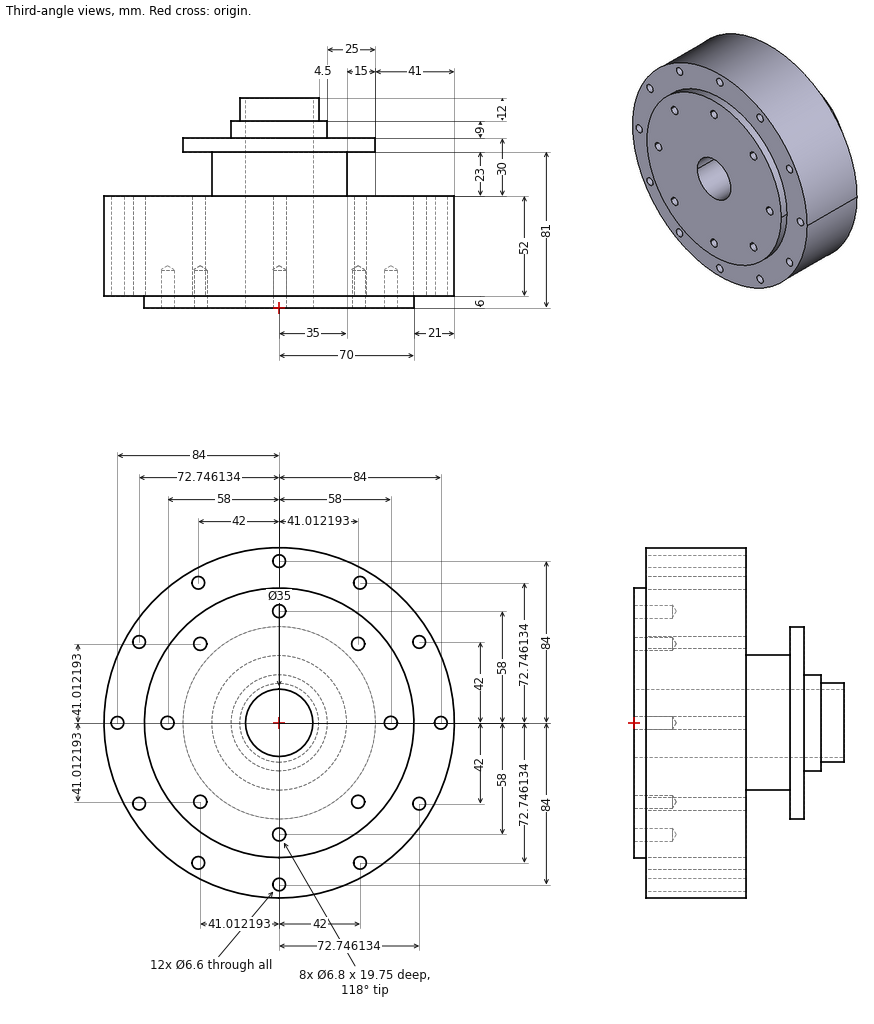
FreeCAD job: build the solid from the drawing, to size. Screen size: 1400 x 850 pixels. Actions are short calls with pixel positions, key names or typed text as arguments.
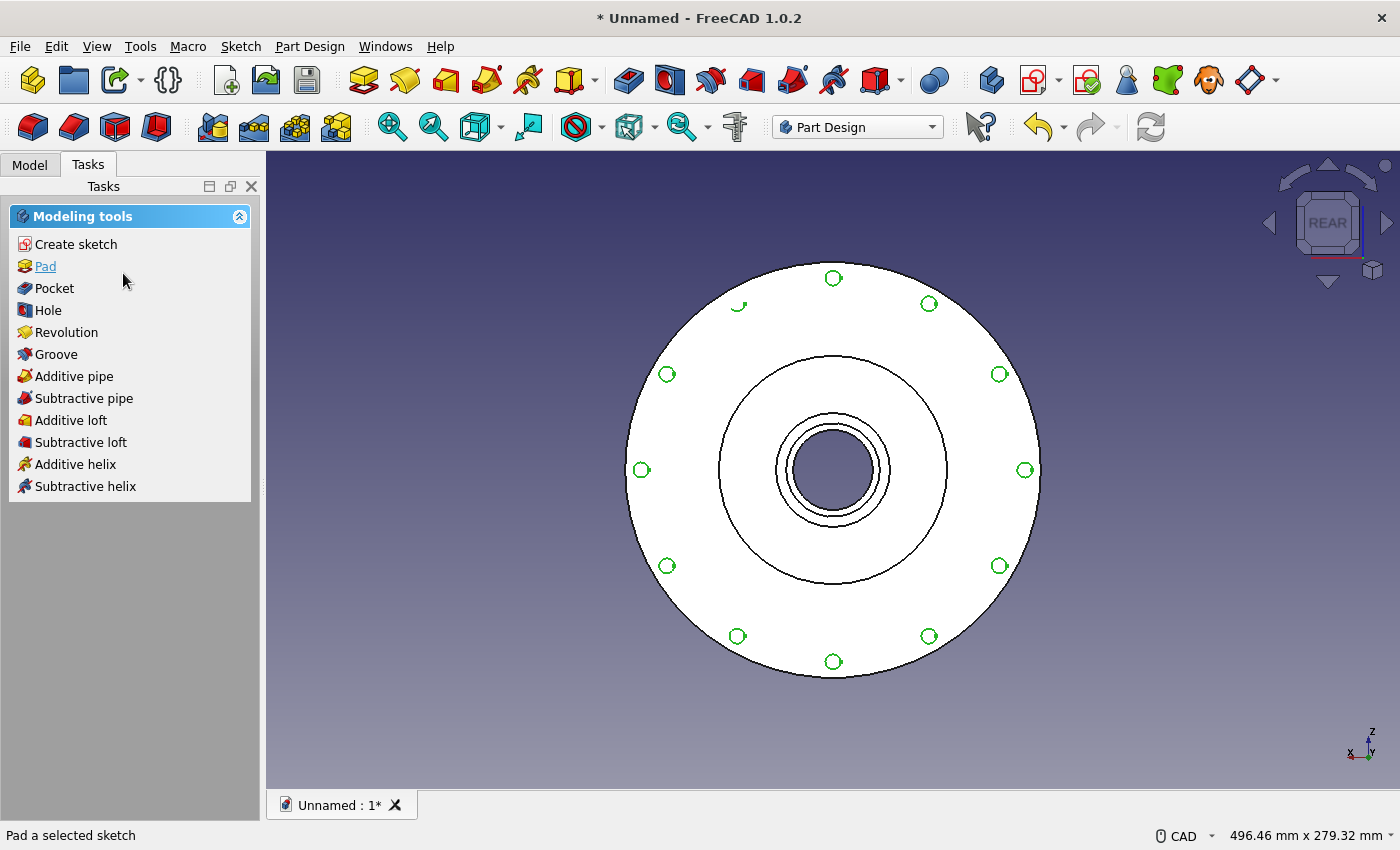
click(670, 80)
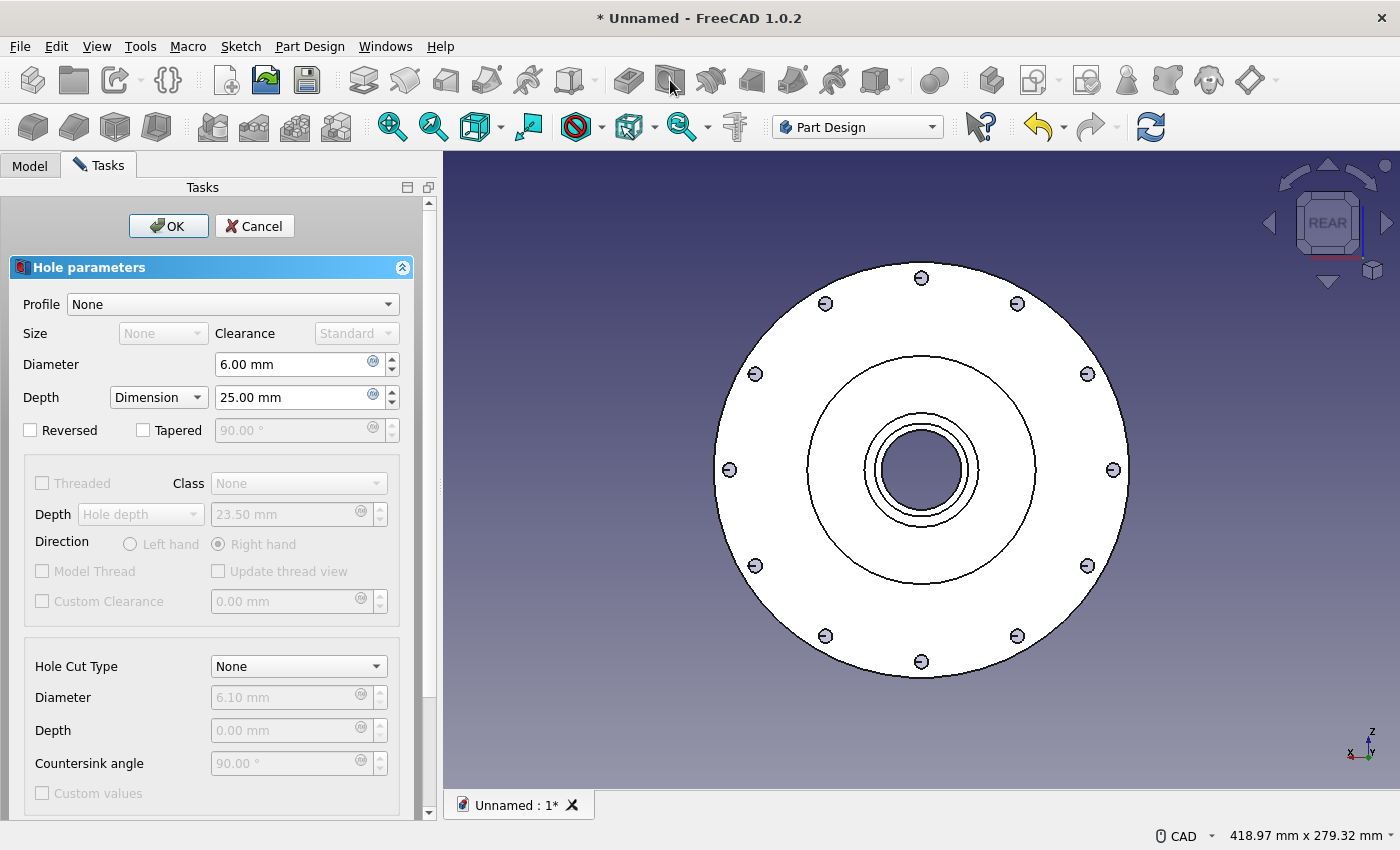
triple_click(300, 364)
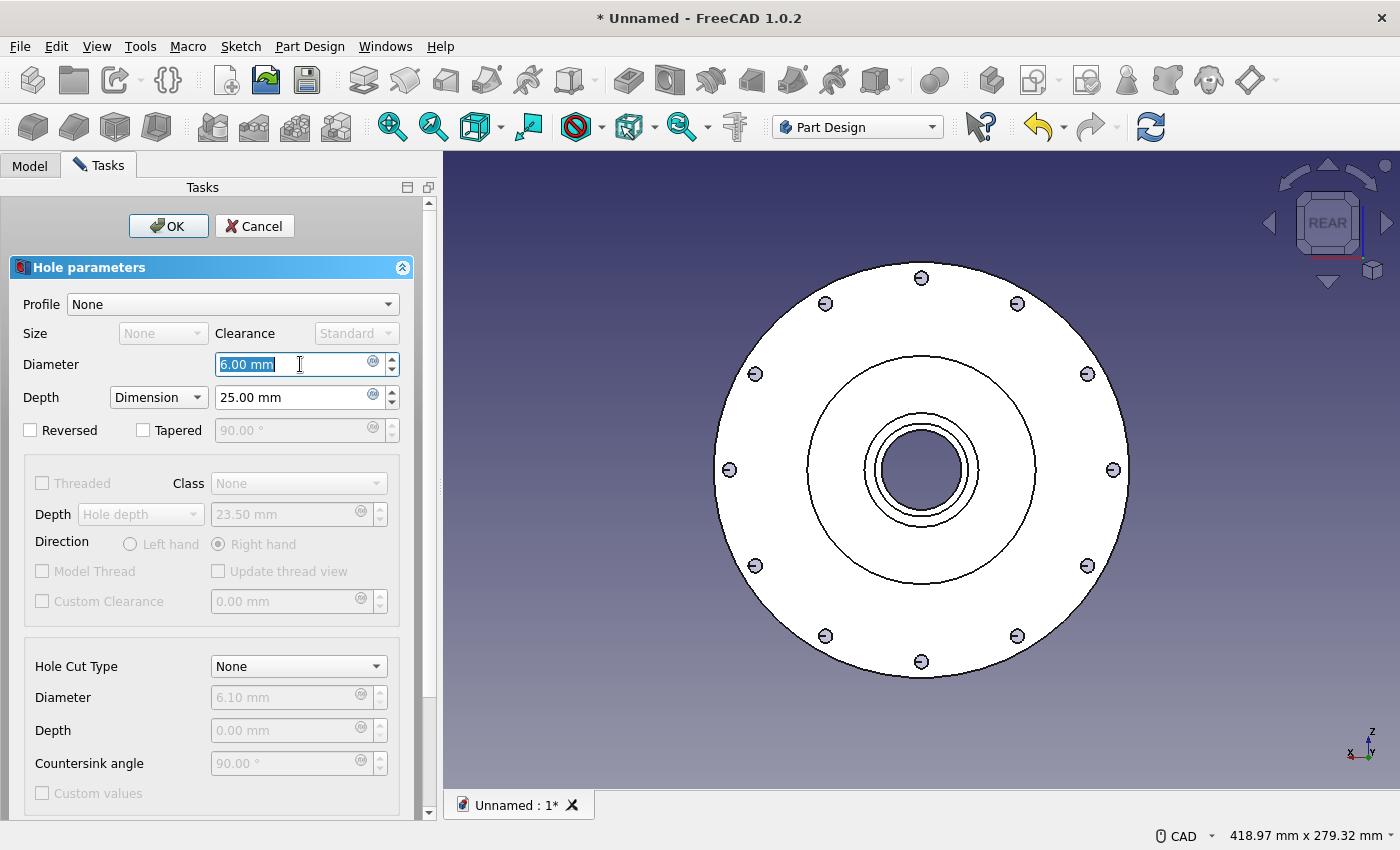
text(6.6)
key(Tab)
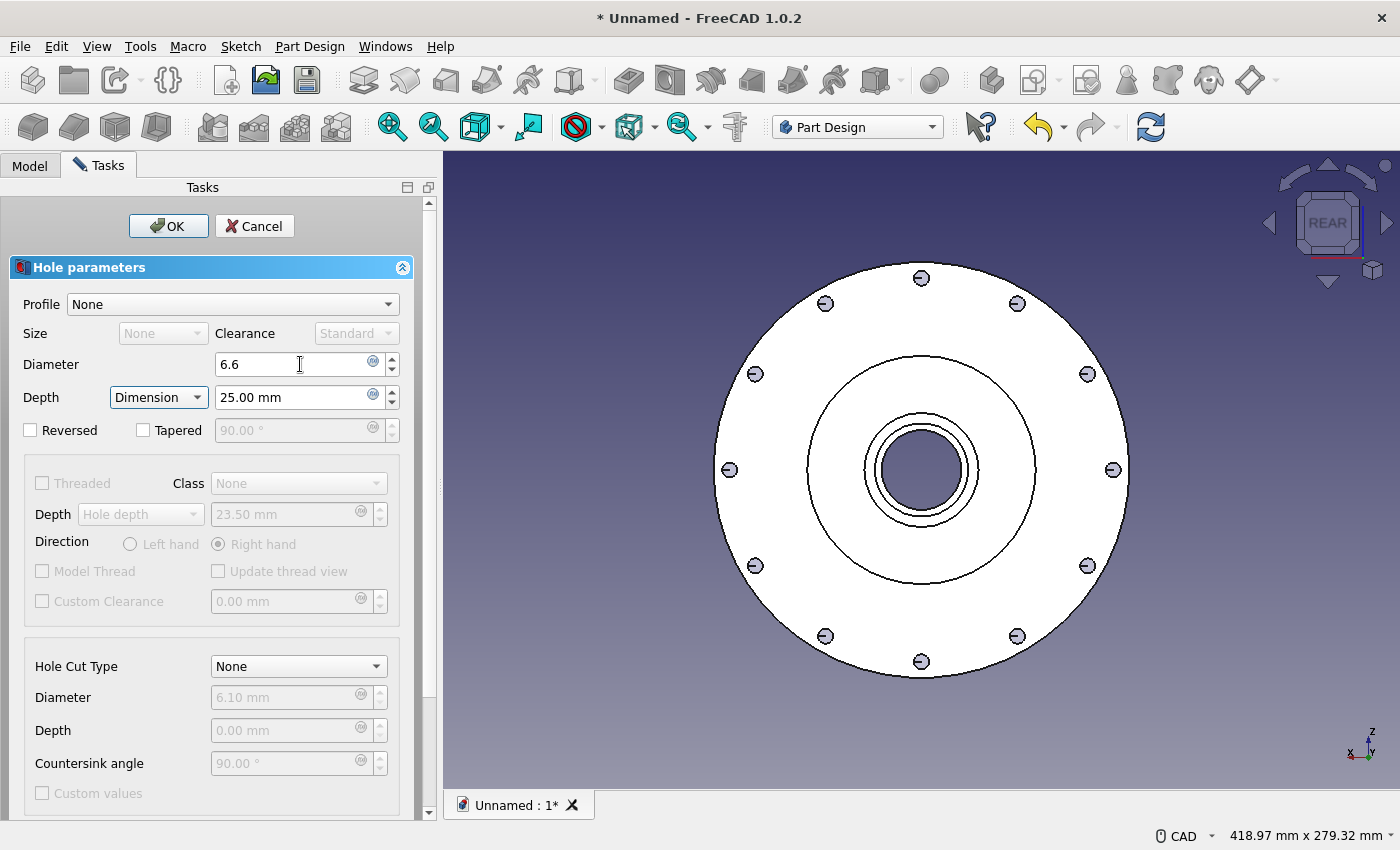
click(160, 398)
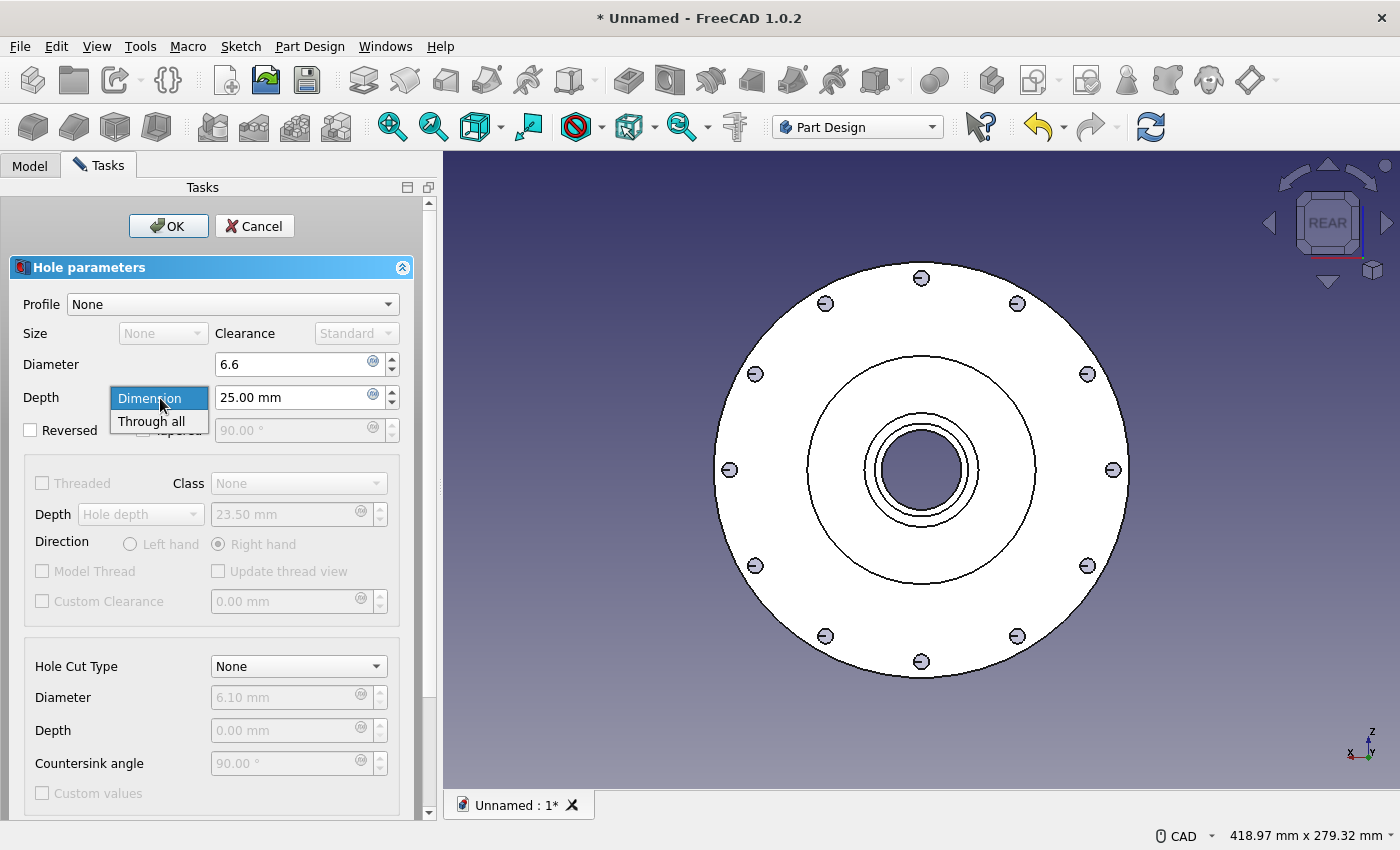
click(158, 422)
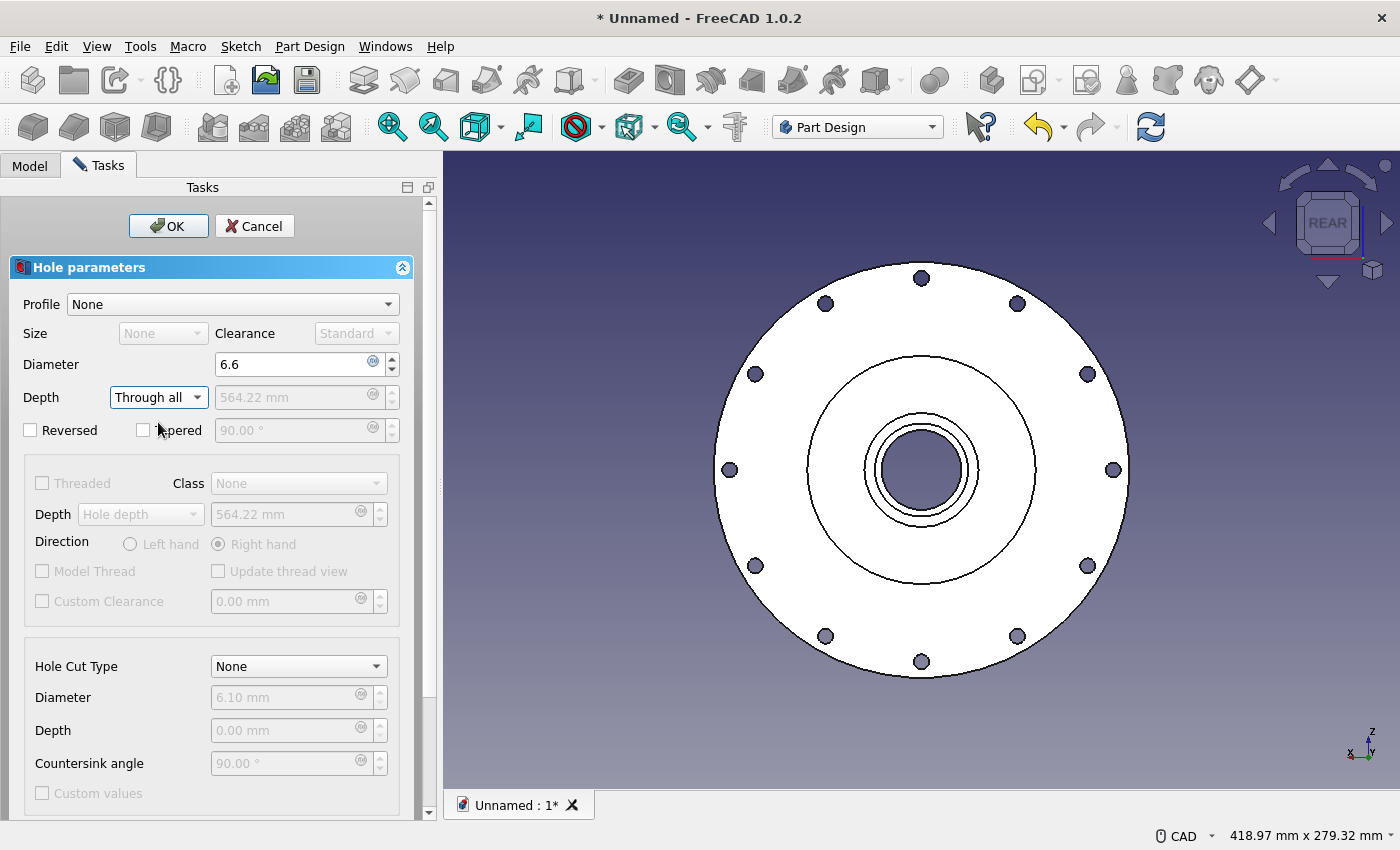
click(169, 226)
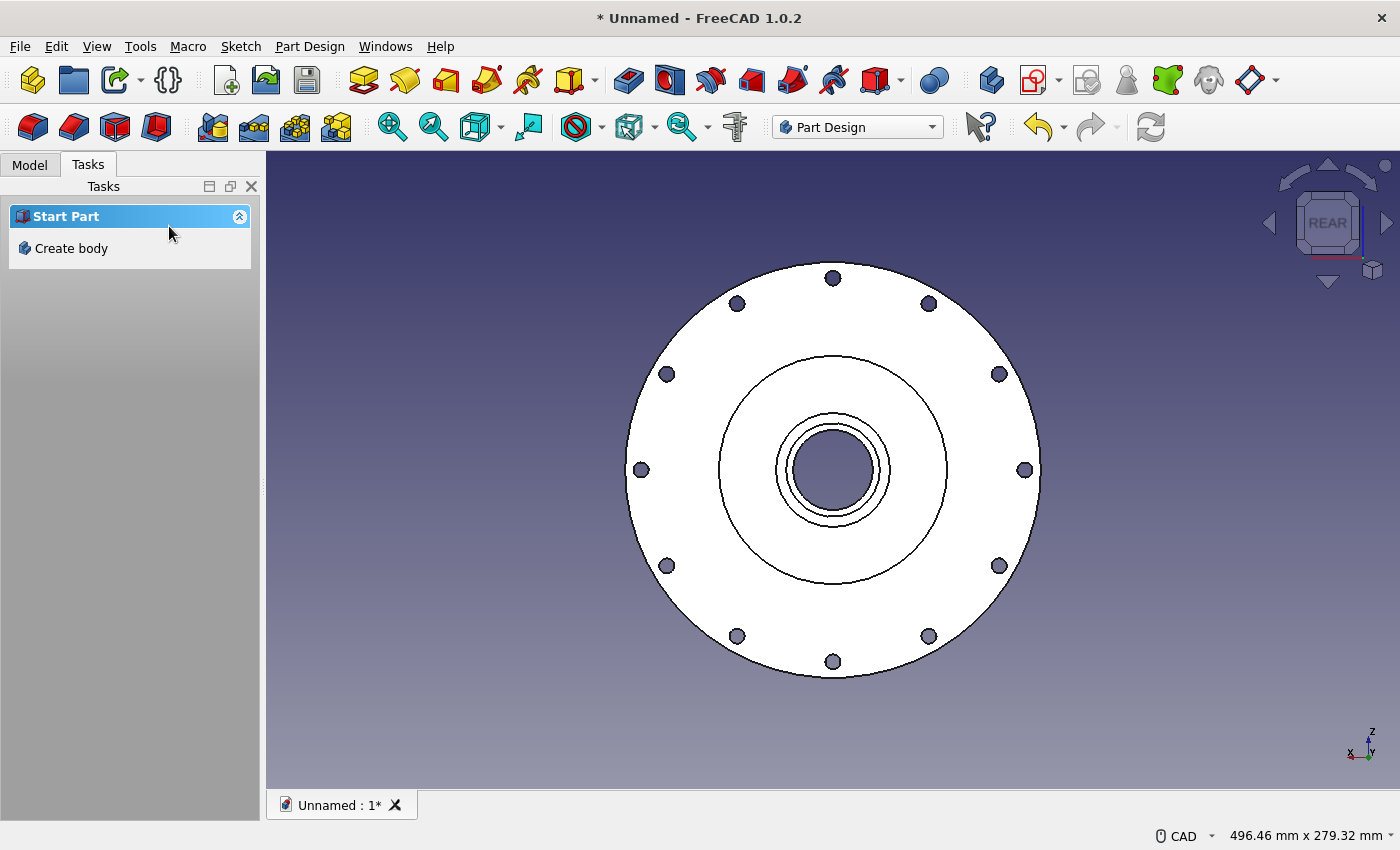
key(0)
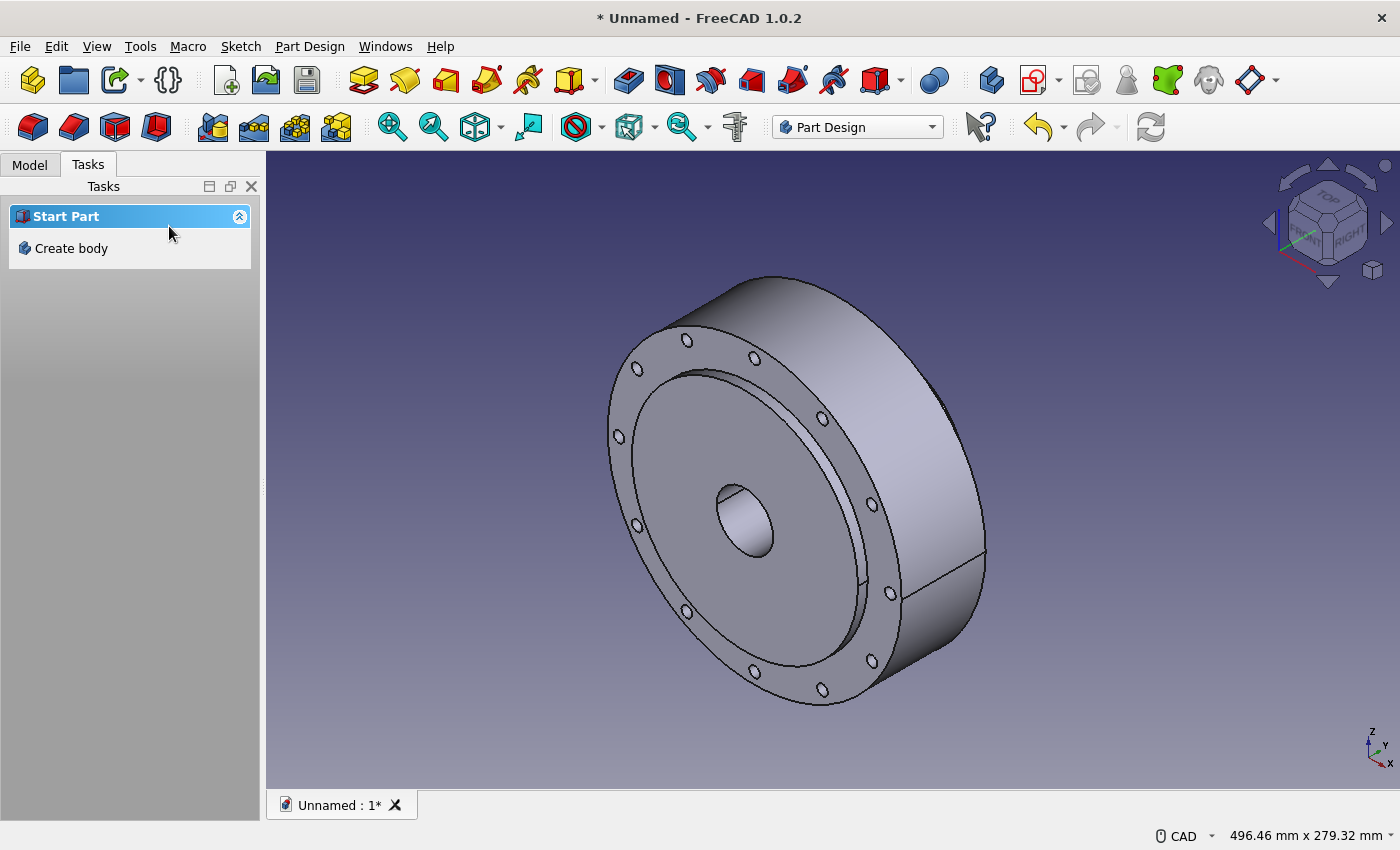
click(777, 464)